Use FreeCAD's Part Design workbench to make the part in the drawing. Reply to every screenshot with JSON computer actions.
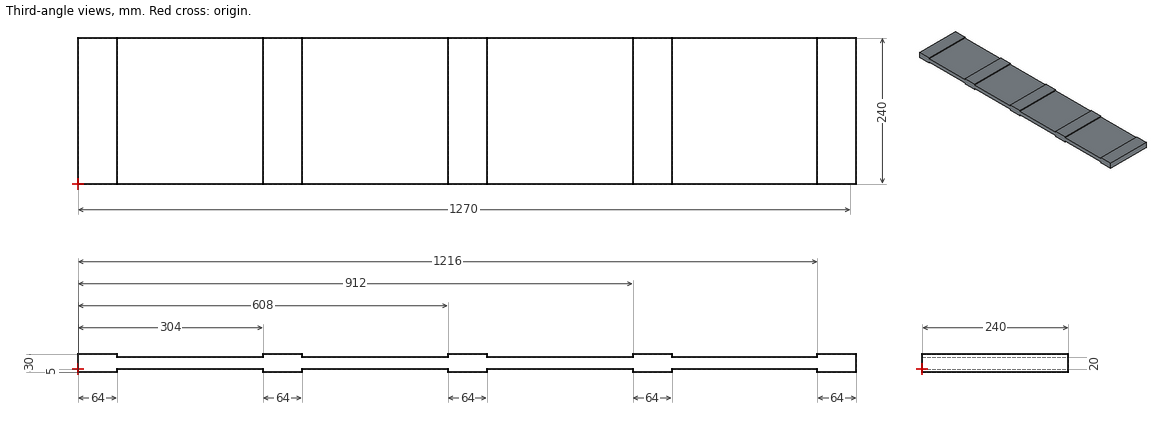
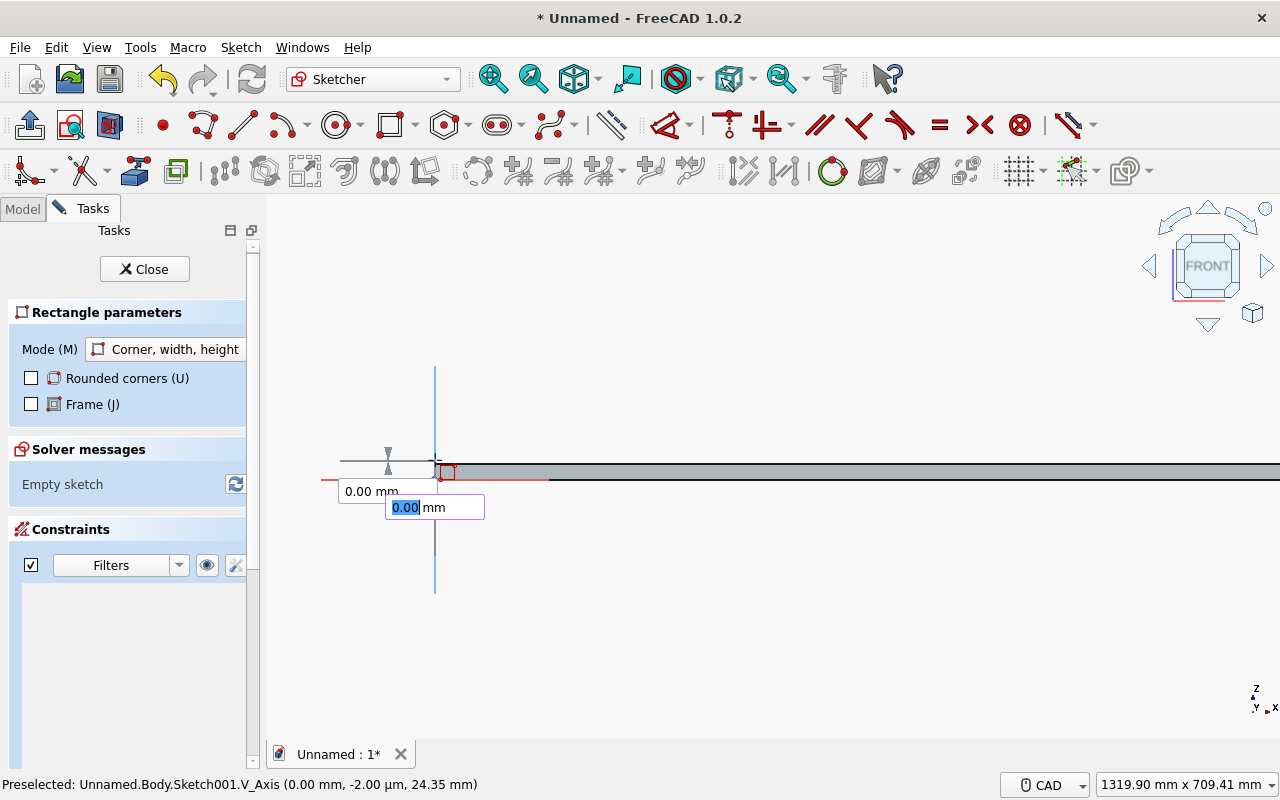
{"action": "scroll", "coordinate": [484, 484], "scroll_direction": "up", "scroll_amount": 8}
{"action": "mouse_move", "coordinate": [484, 480]}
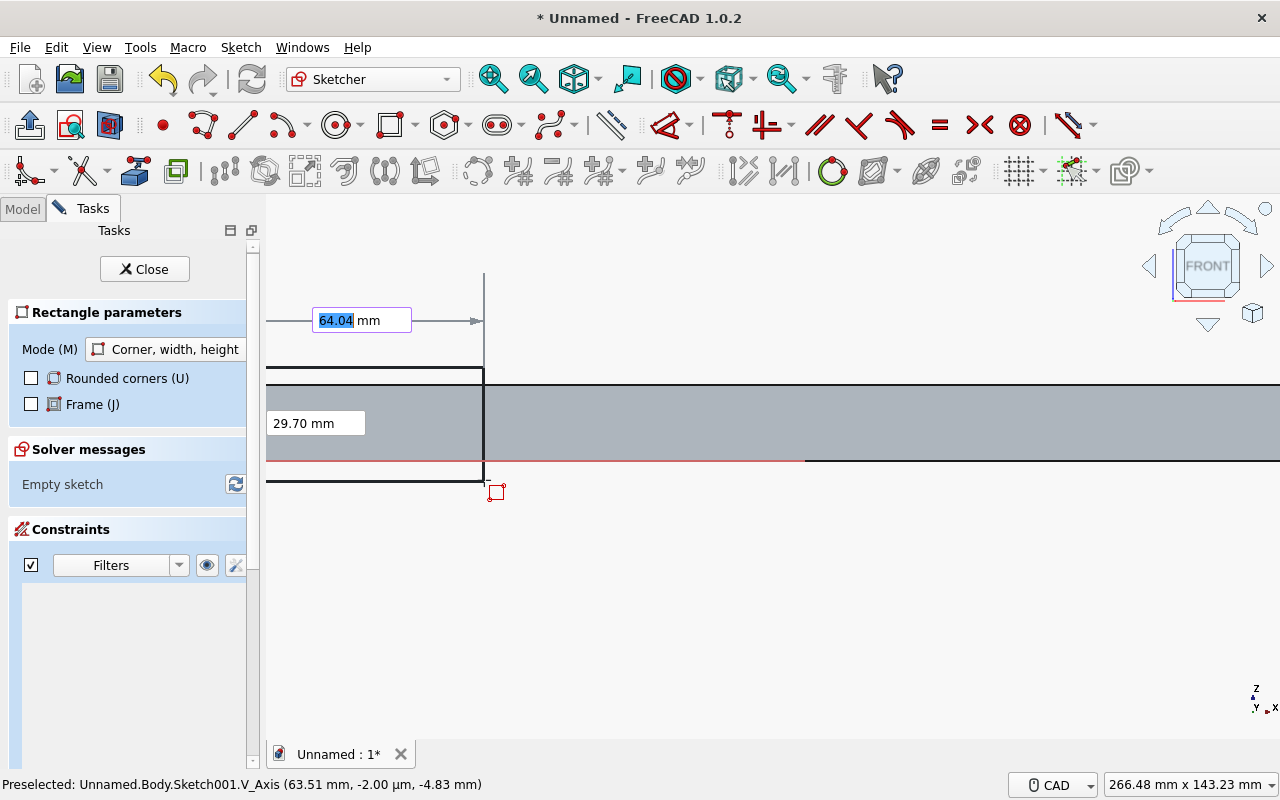
{"action": "type", "text": "64"}
{"action": "key", "text": "Tab"}
{"action": "type", "text": "30"}
{"action": "key", "text": "Return"}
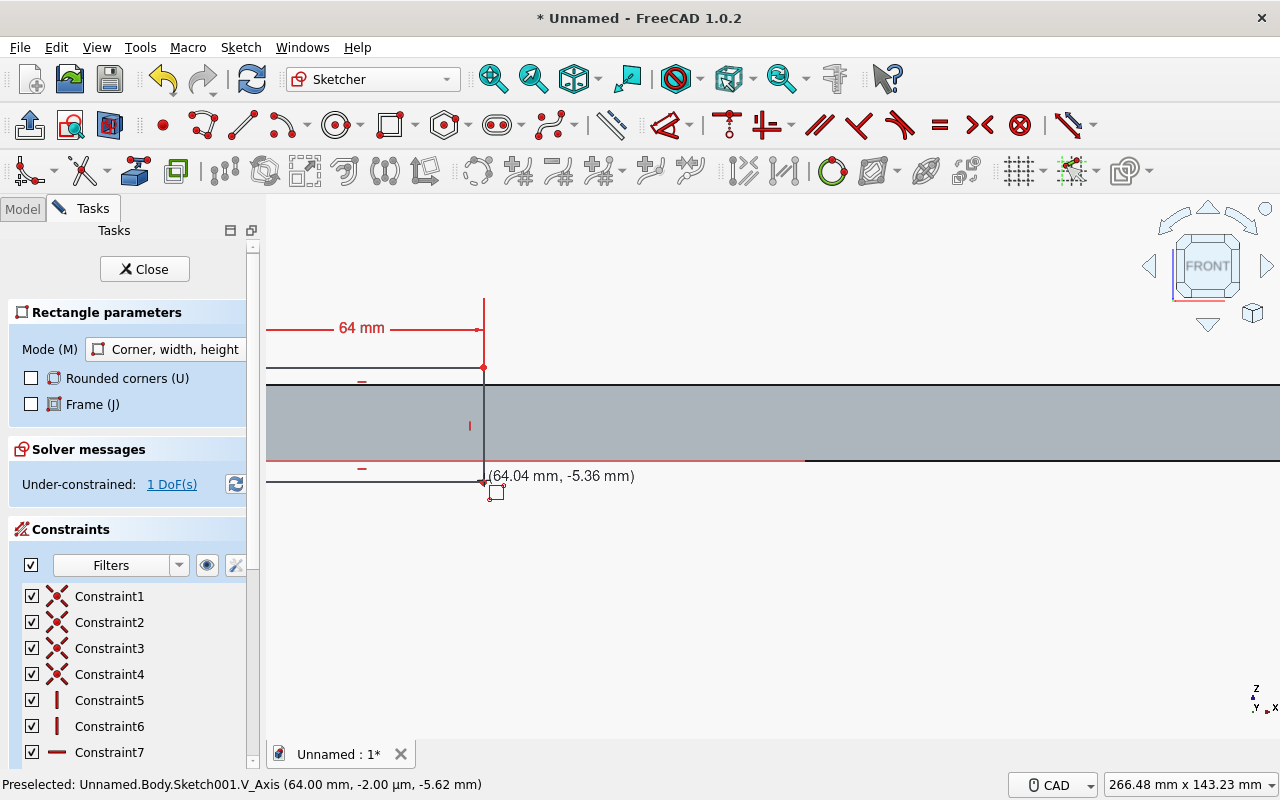
{"action": "scroll", "coordinate": [459, 472], "scroll_direction": "down", "scroll_amount": 11}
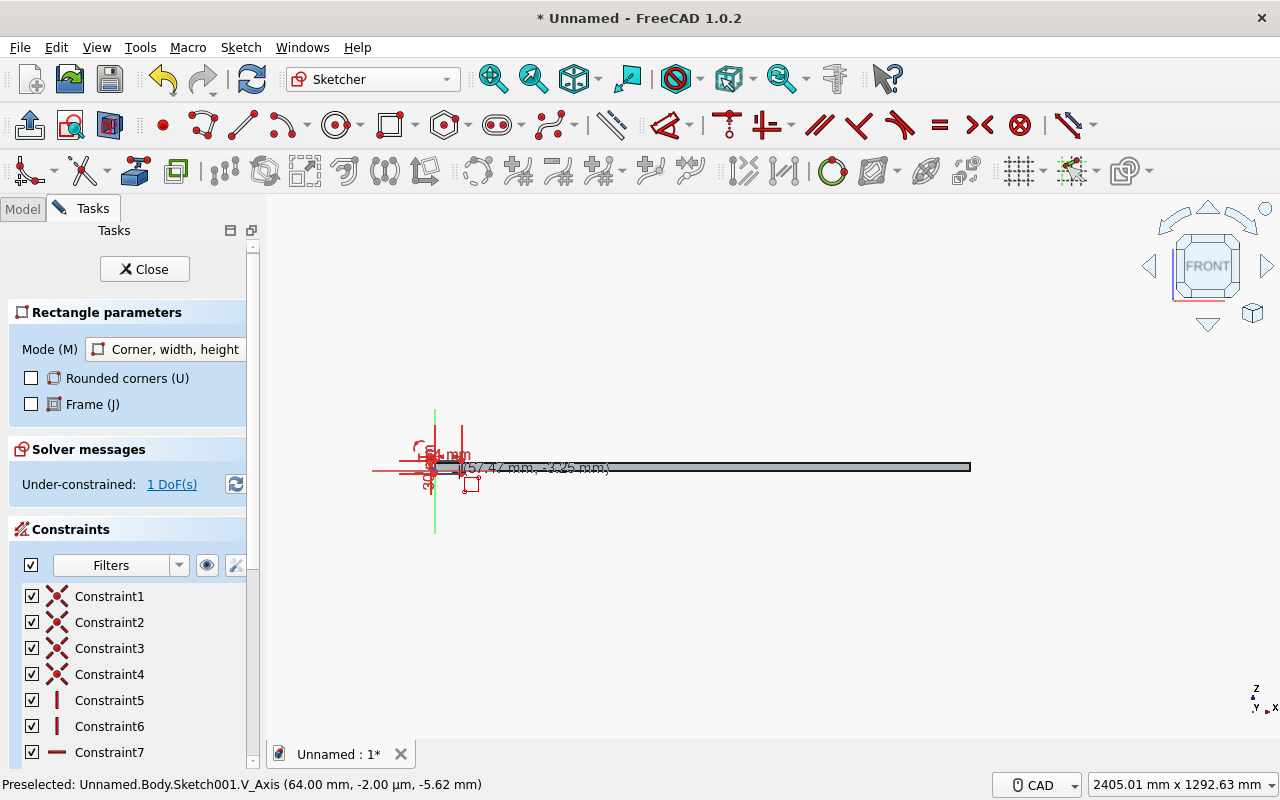
{"action": "scroll", "coordinate": [563, 461], "scroll_direction": "up", "scroll_amount": 3}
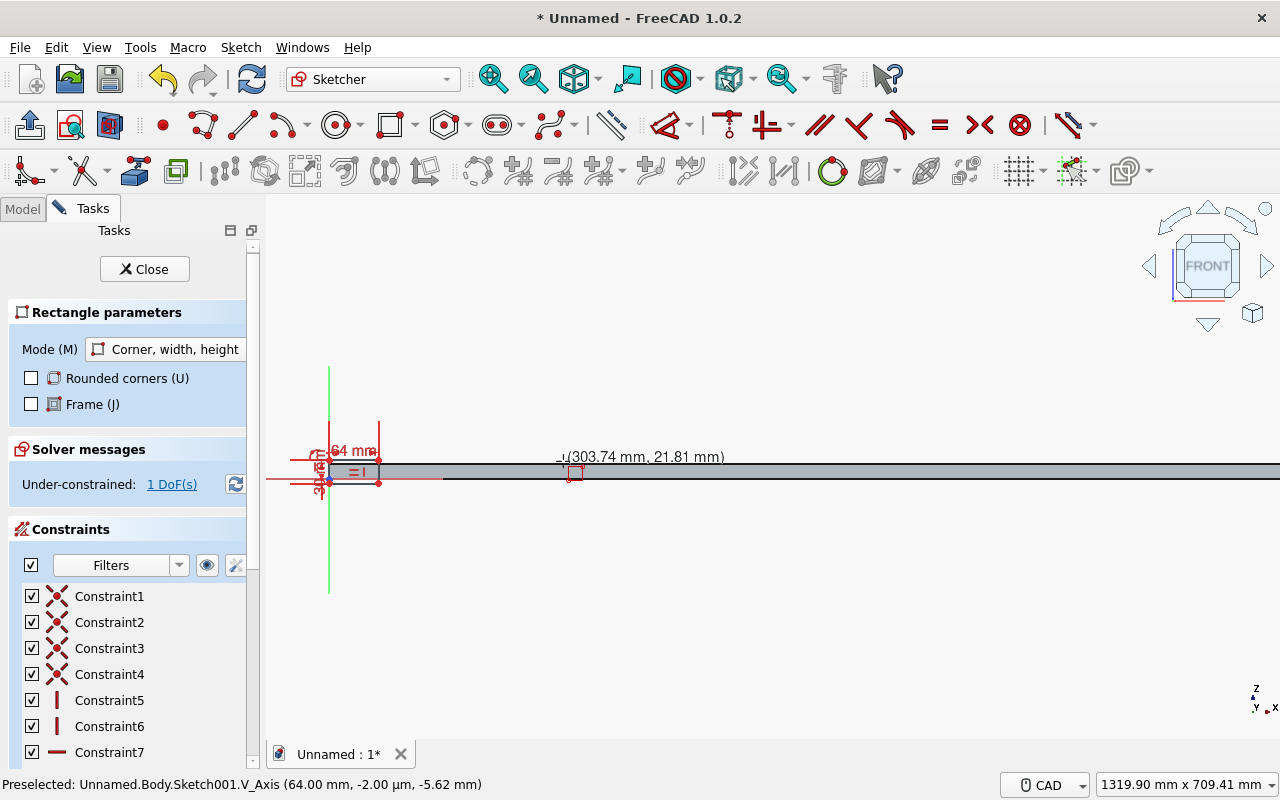
{"action": "left_click", "coordinate": [563, 460]}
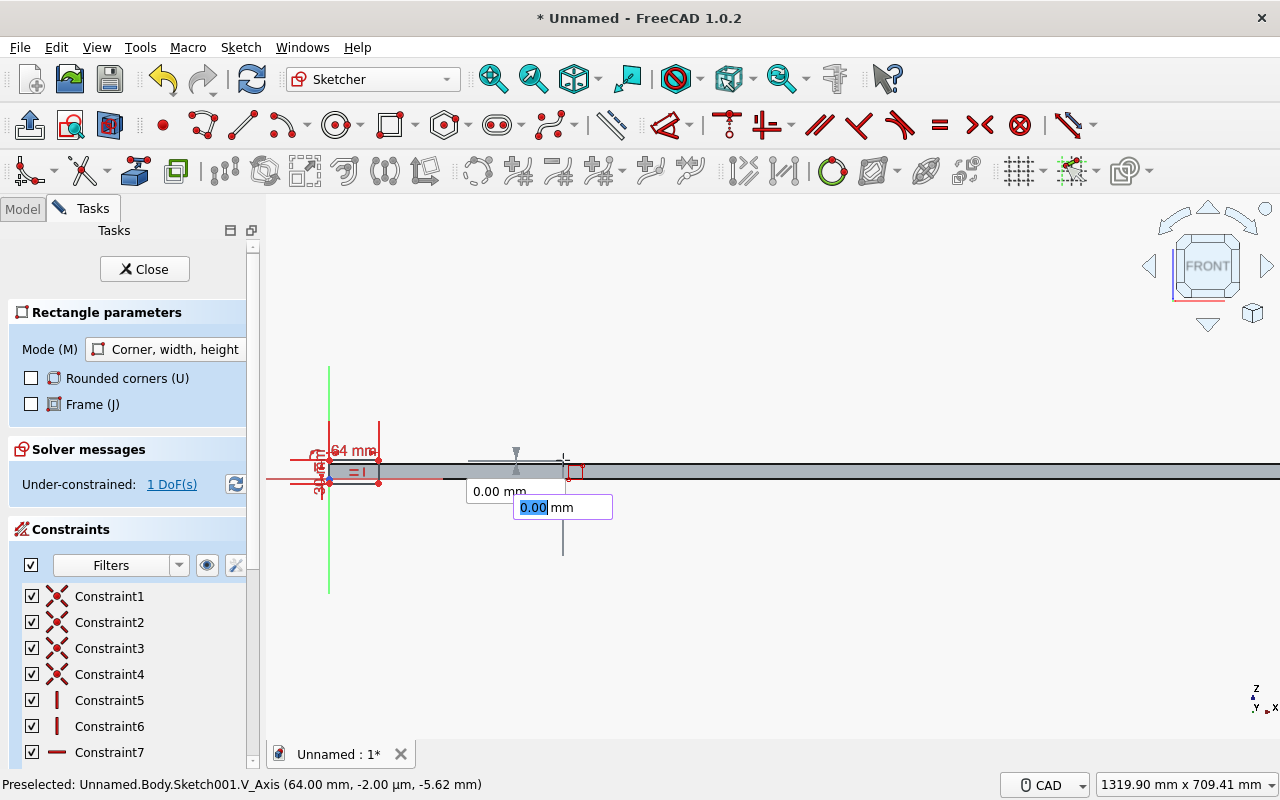
{"action": "scroll", "coordinate": [612, 483], "scroll_direction": "up", "scroll_amount": 8}
{"action": "mouse_move", "coordinate": [611, 481]}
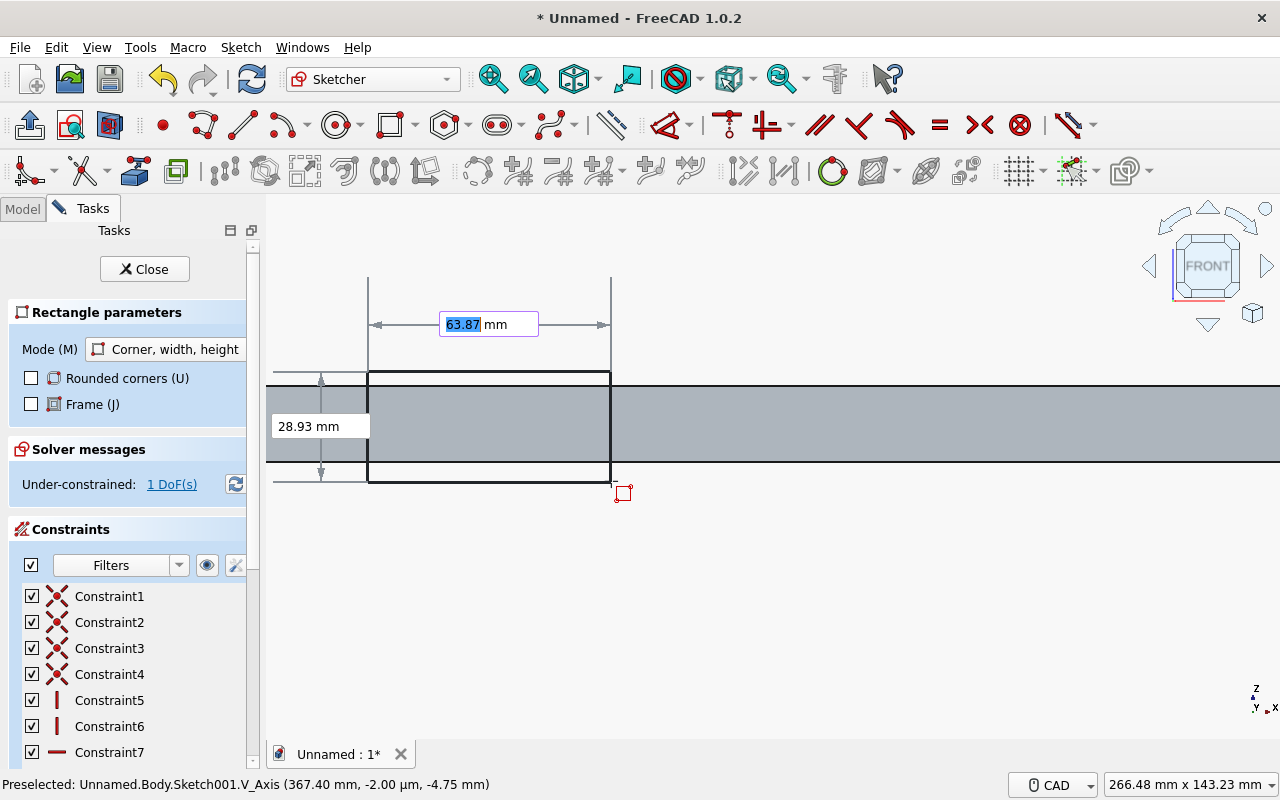
{"action": "type", "text": "64"}
{"action": "key", "text": "Tab"}
{"action": "type", "text": "30"}
{"action": "key", "text": "Return"}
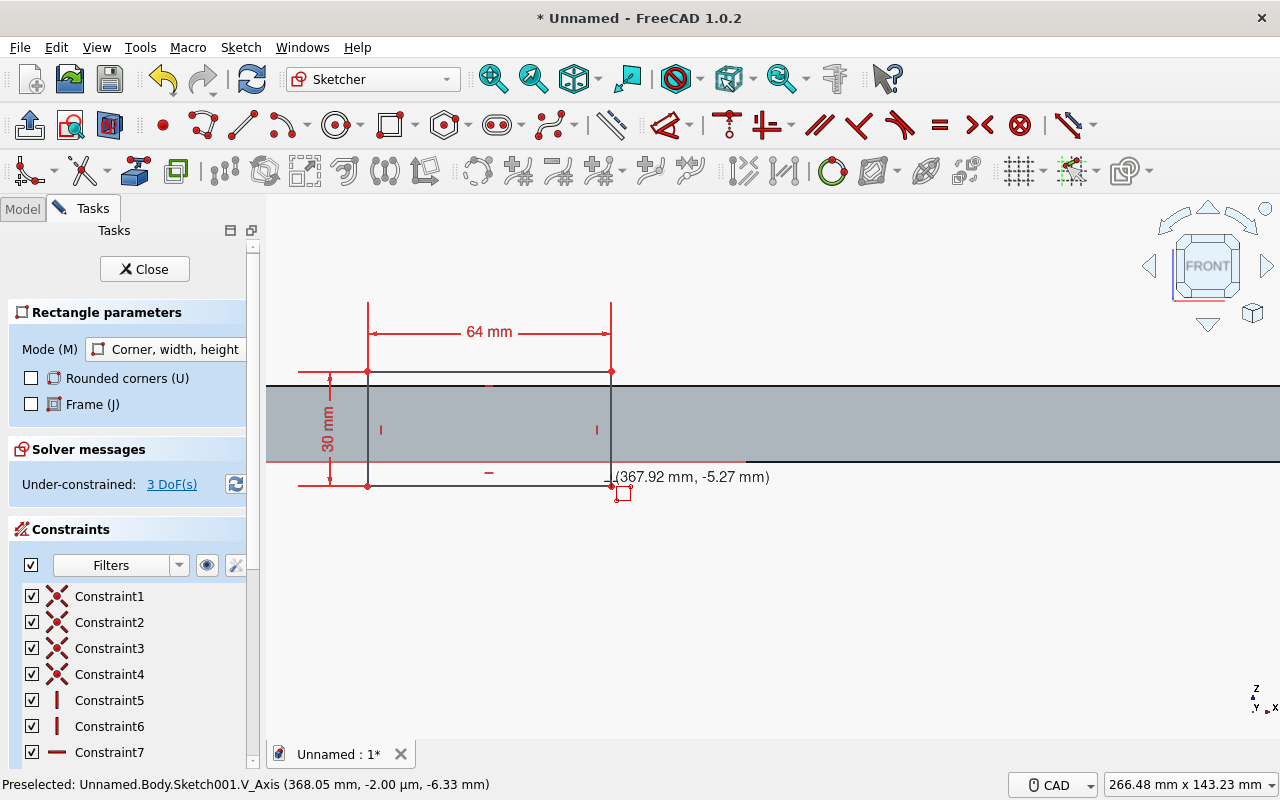
{"action": "scroll", "coordinate": [587, 472], "scroll_direction": "down", "scroll_amount": 11}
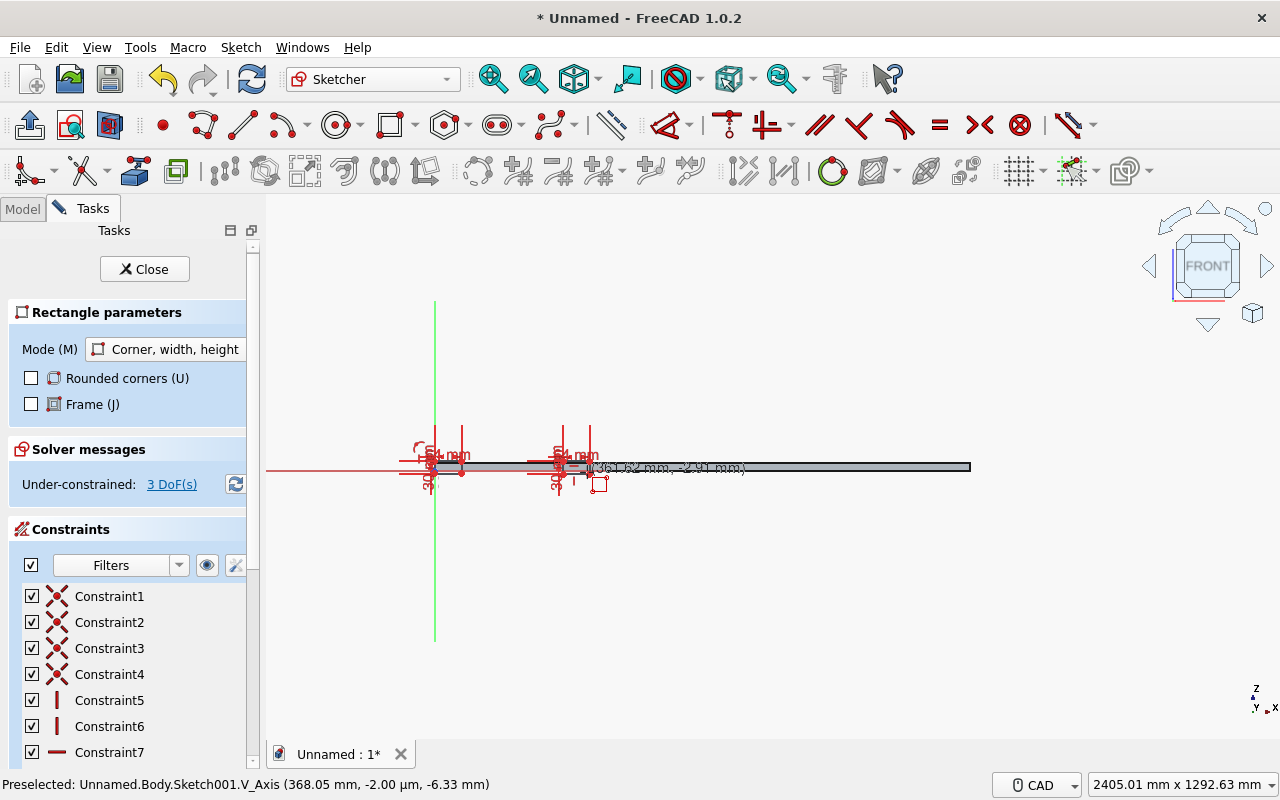
{"action": "scroll", "coordinate": [691, 461], "scroll_direction": "up", "scroll_amount": 3}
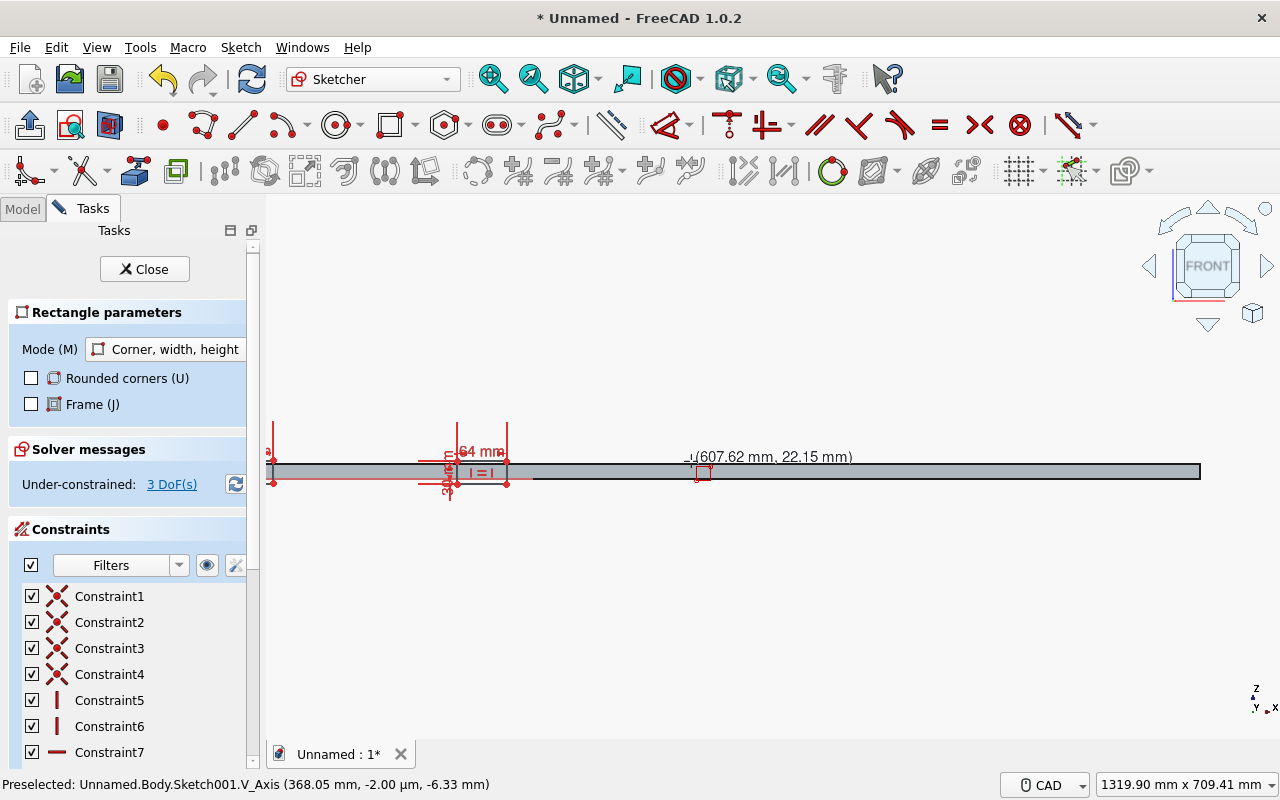
{"action": "left_click", "coordinate": [691, 460]}